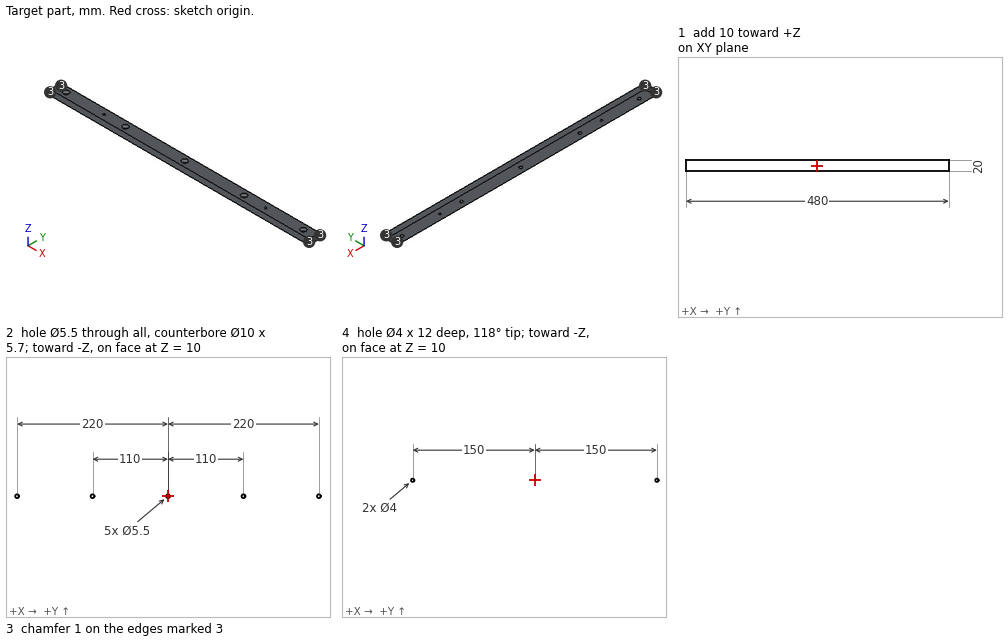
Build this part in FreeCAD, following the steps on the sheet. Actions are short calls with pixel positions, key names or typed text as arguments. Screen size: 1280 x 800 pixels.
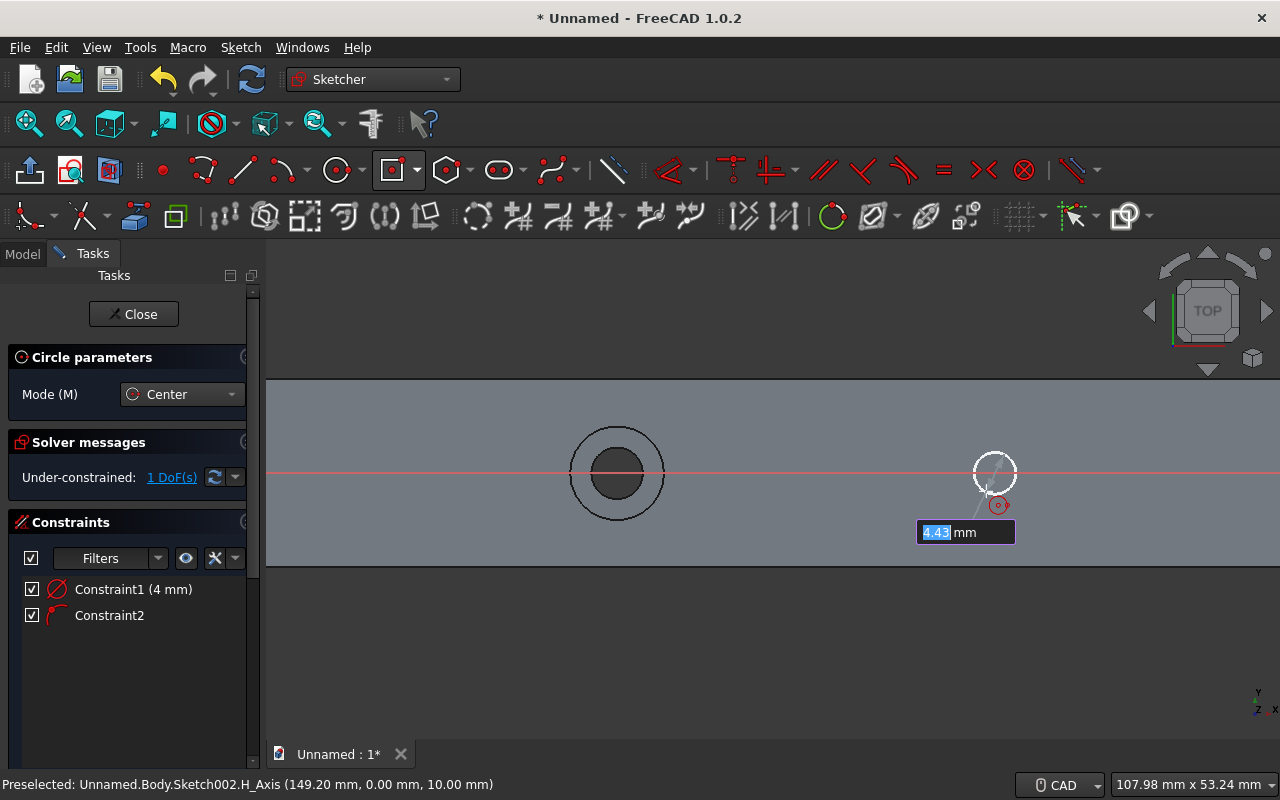
text(4)
key(Return)
key(Escape)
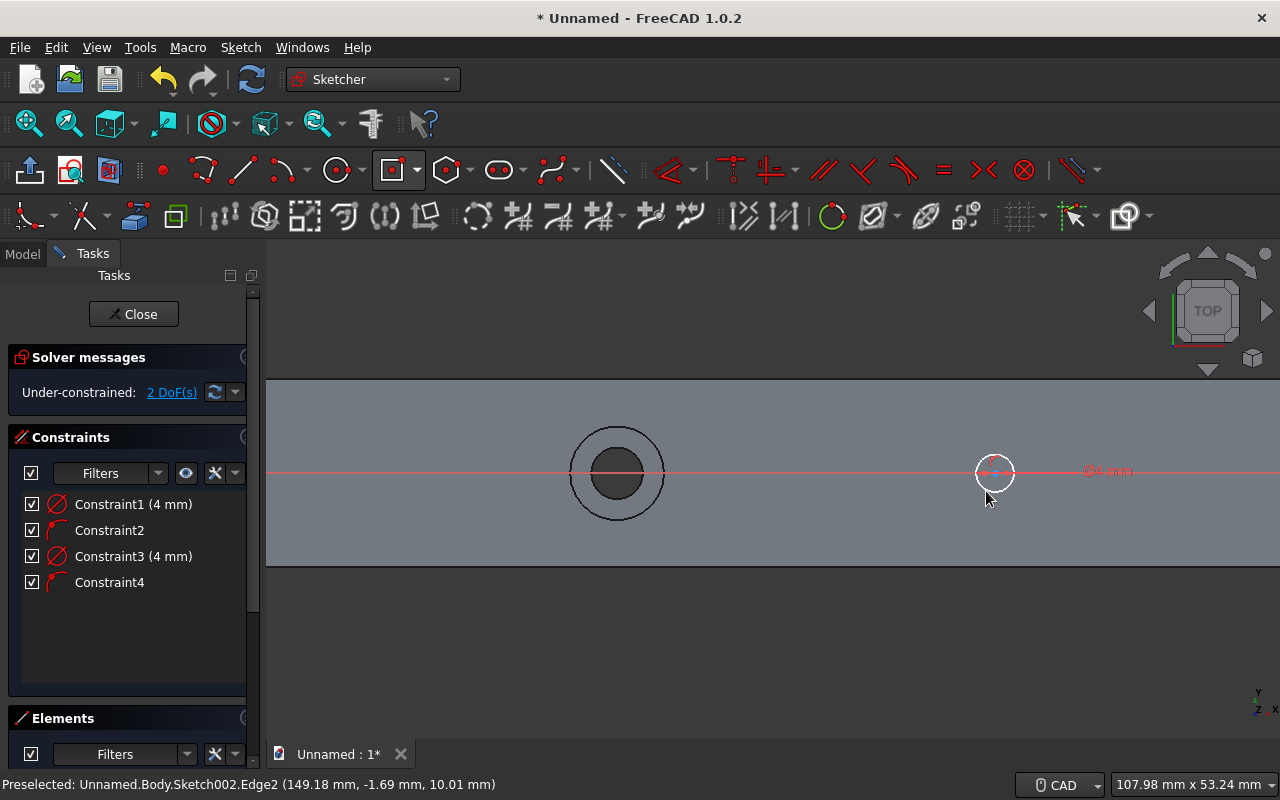
click(668, 170)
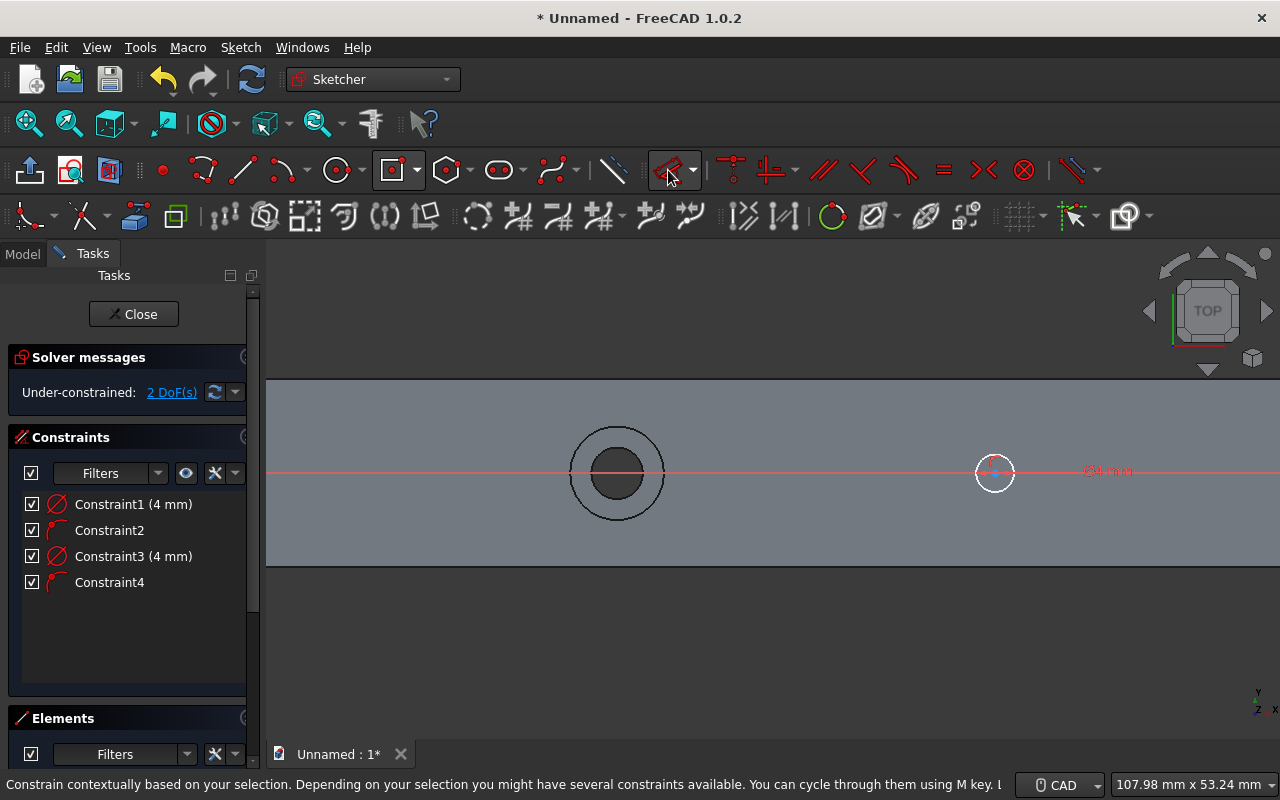
scroll(988, 493, down, 8)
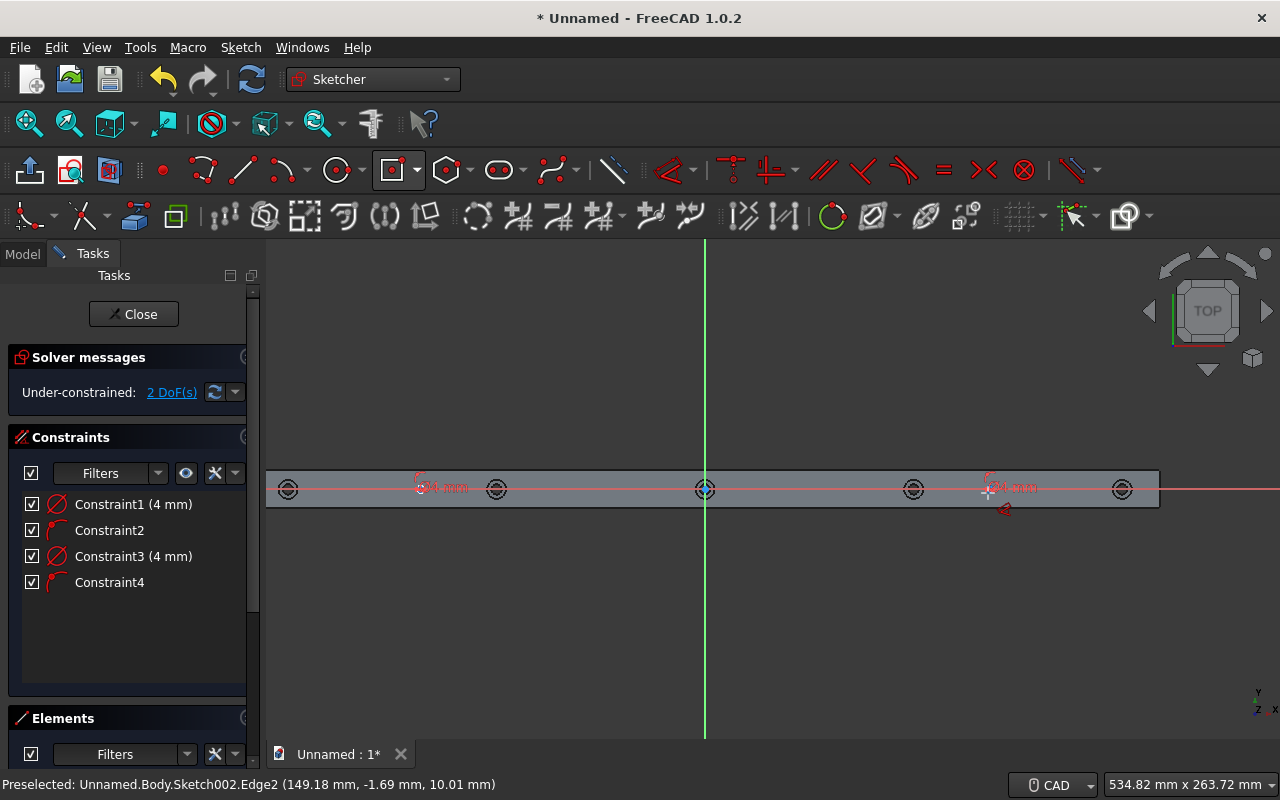
click(421, 489)
click(563, 523)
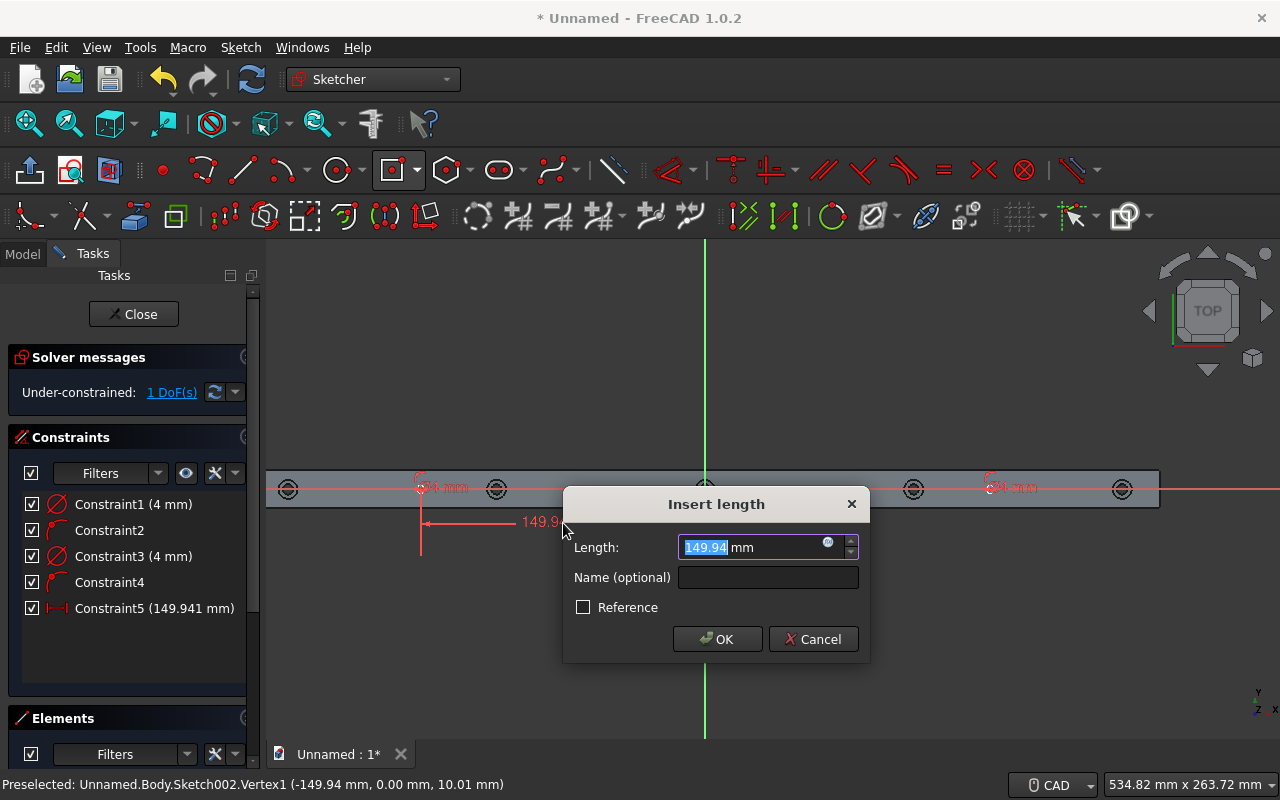
text(150)
key(Return)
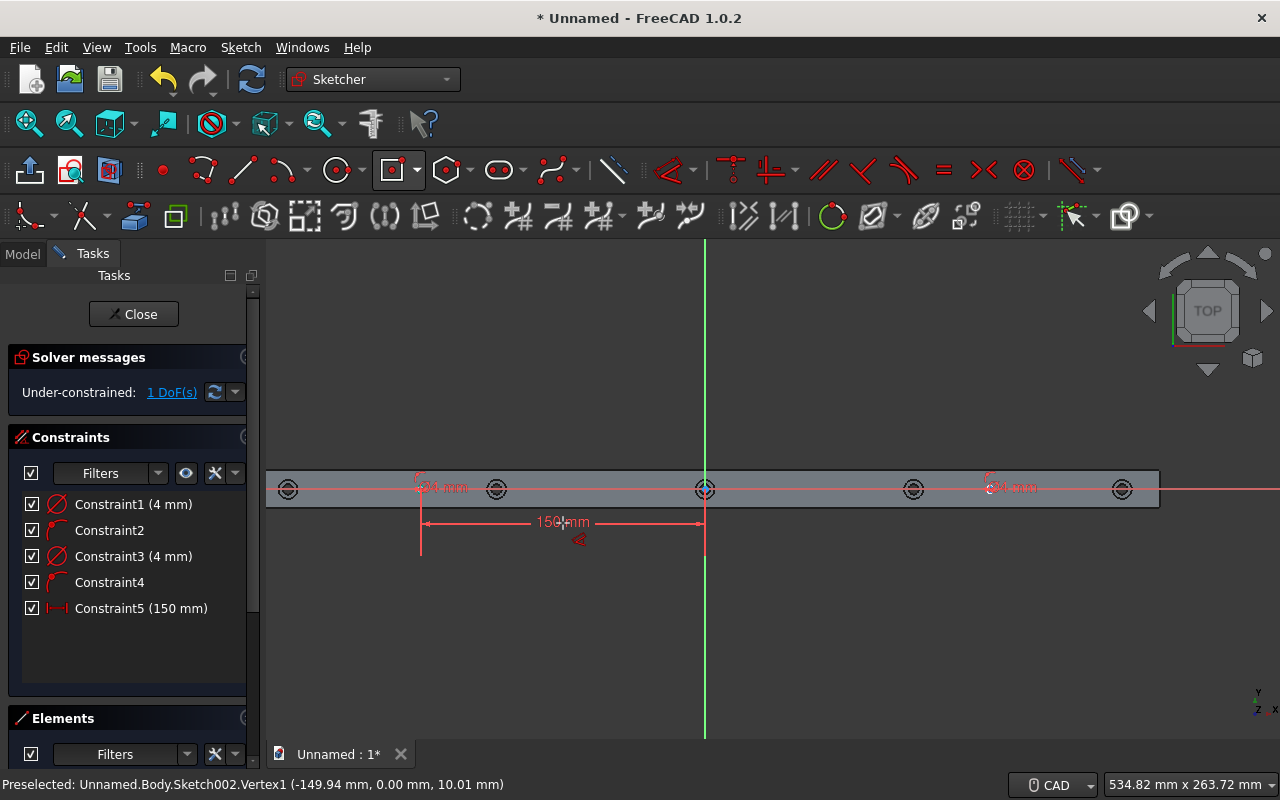
click(990, 489)
click(848, 523)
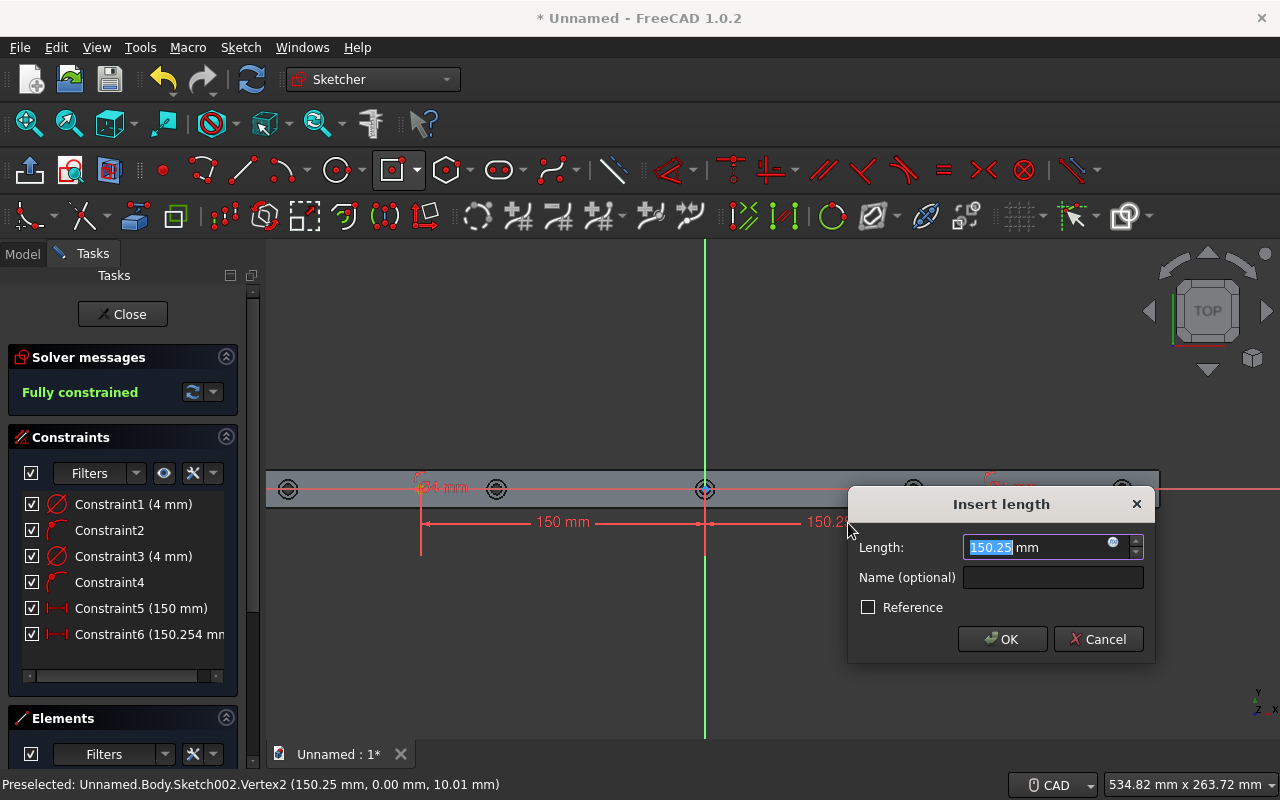
text(150)
key(Return)
key(Escape)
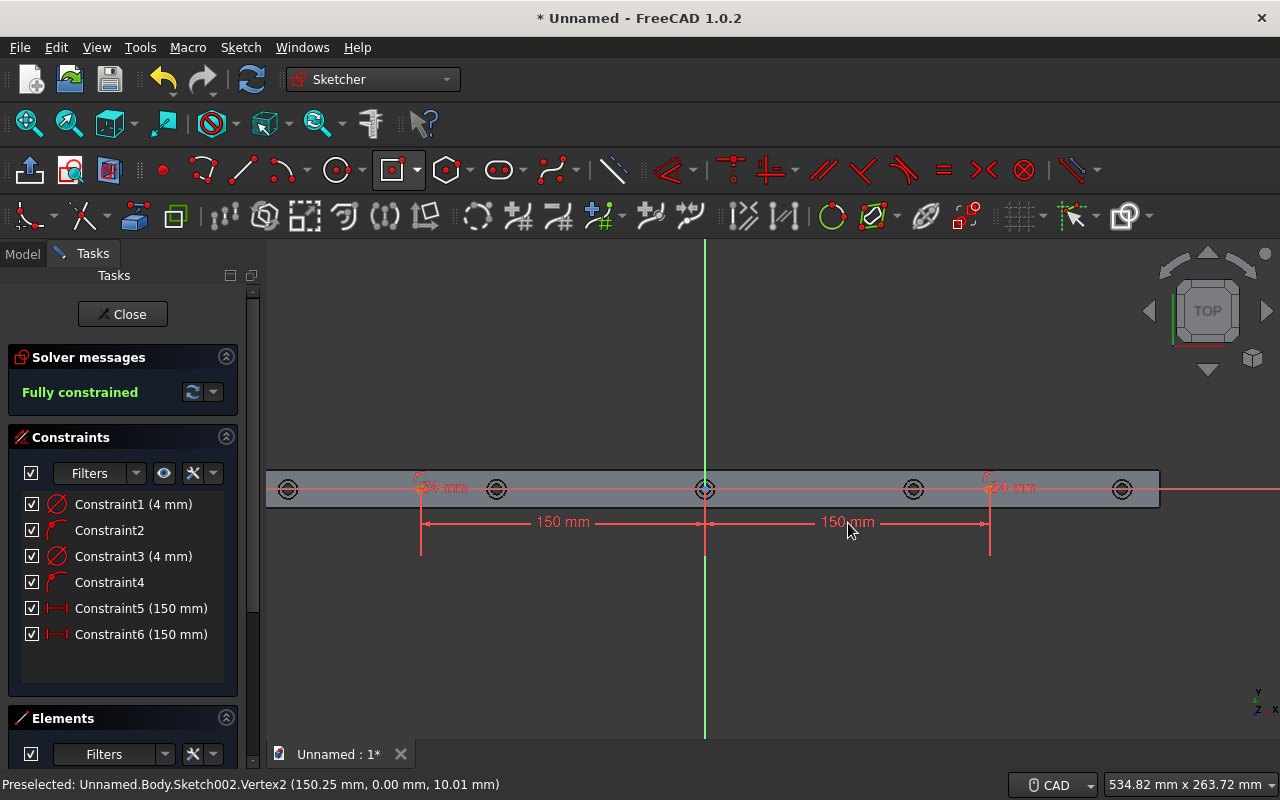
click(123, 314)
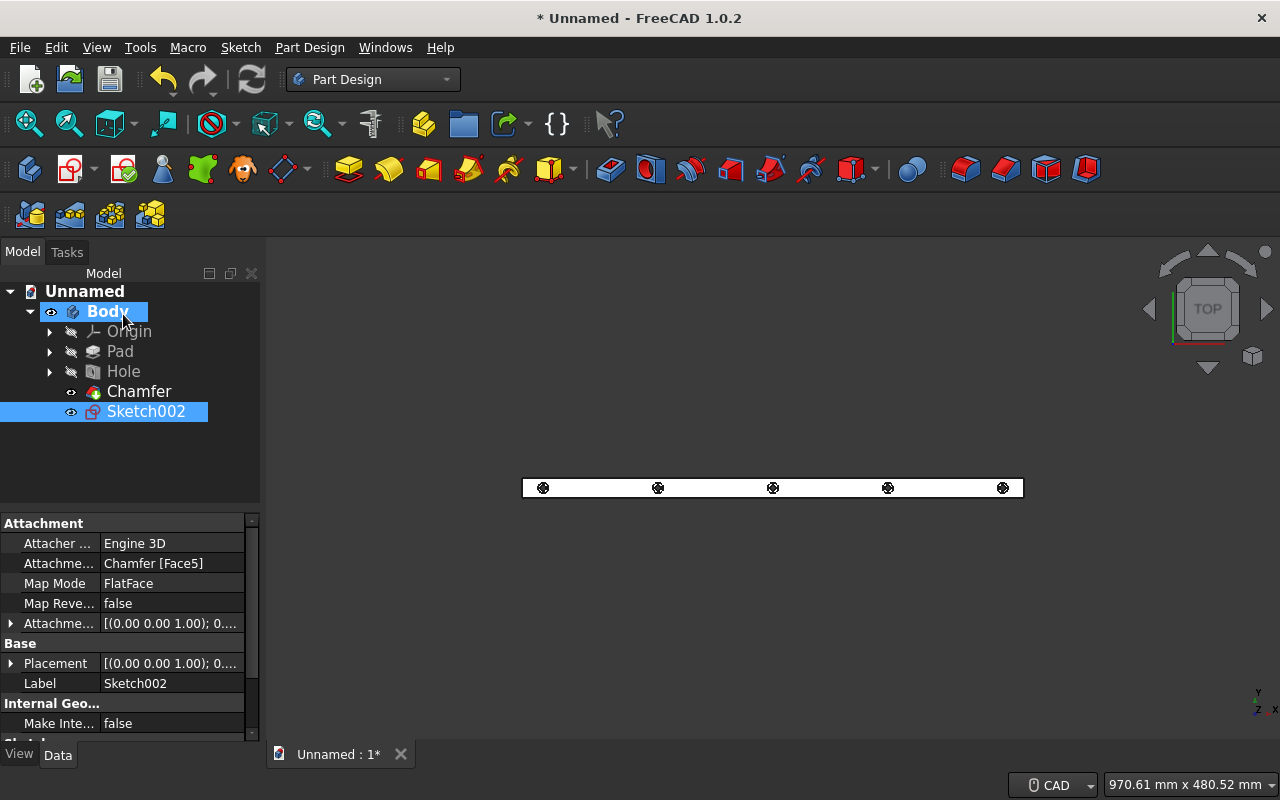
click(652, 170)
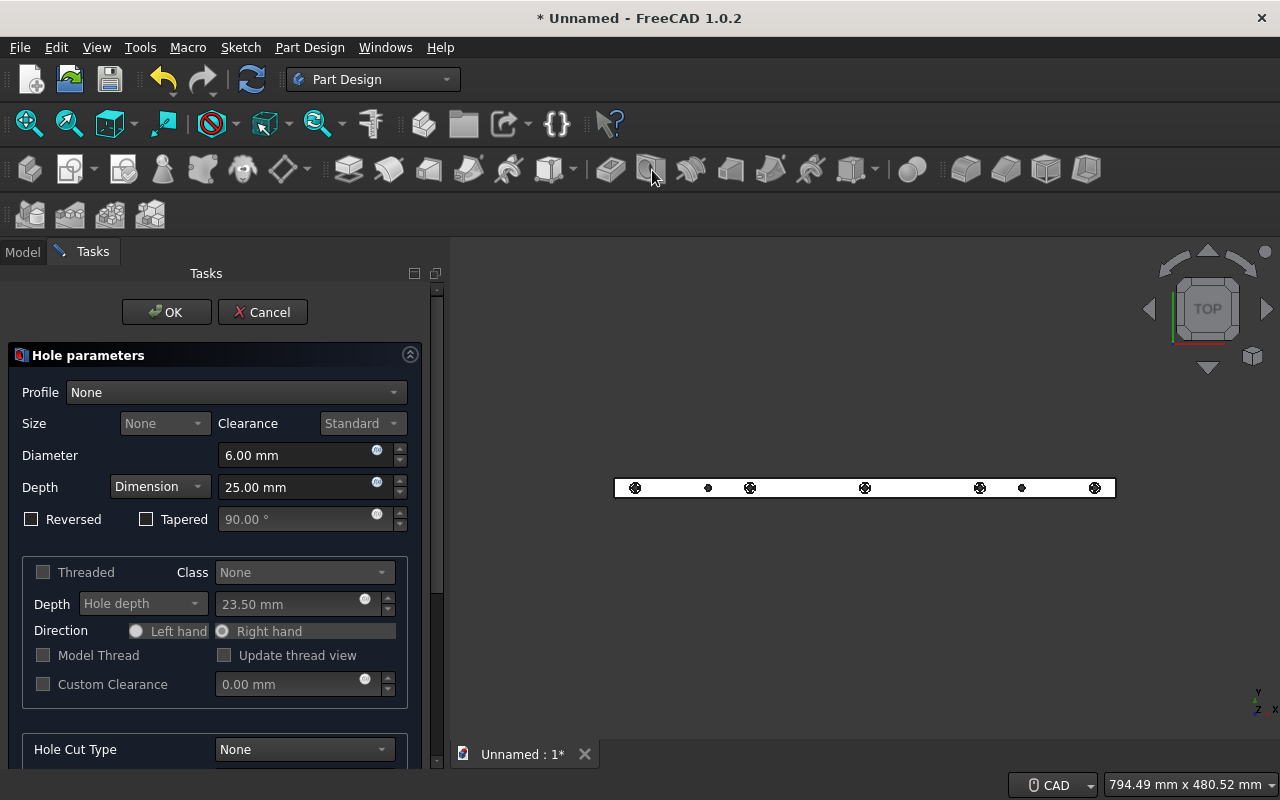
triple_click(305, 455)